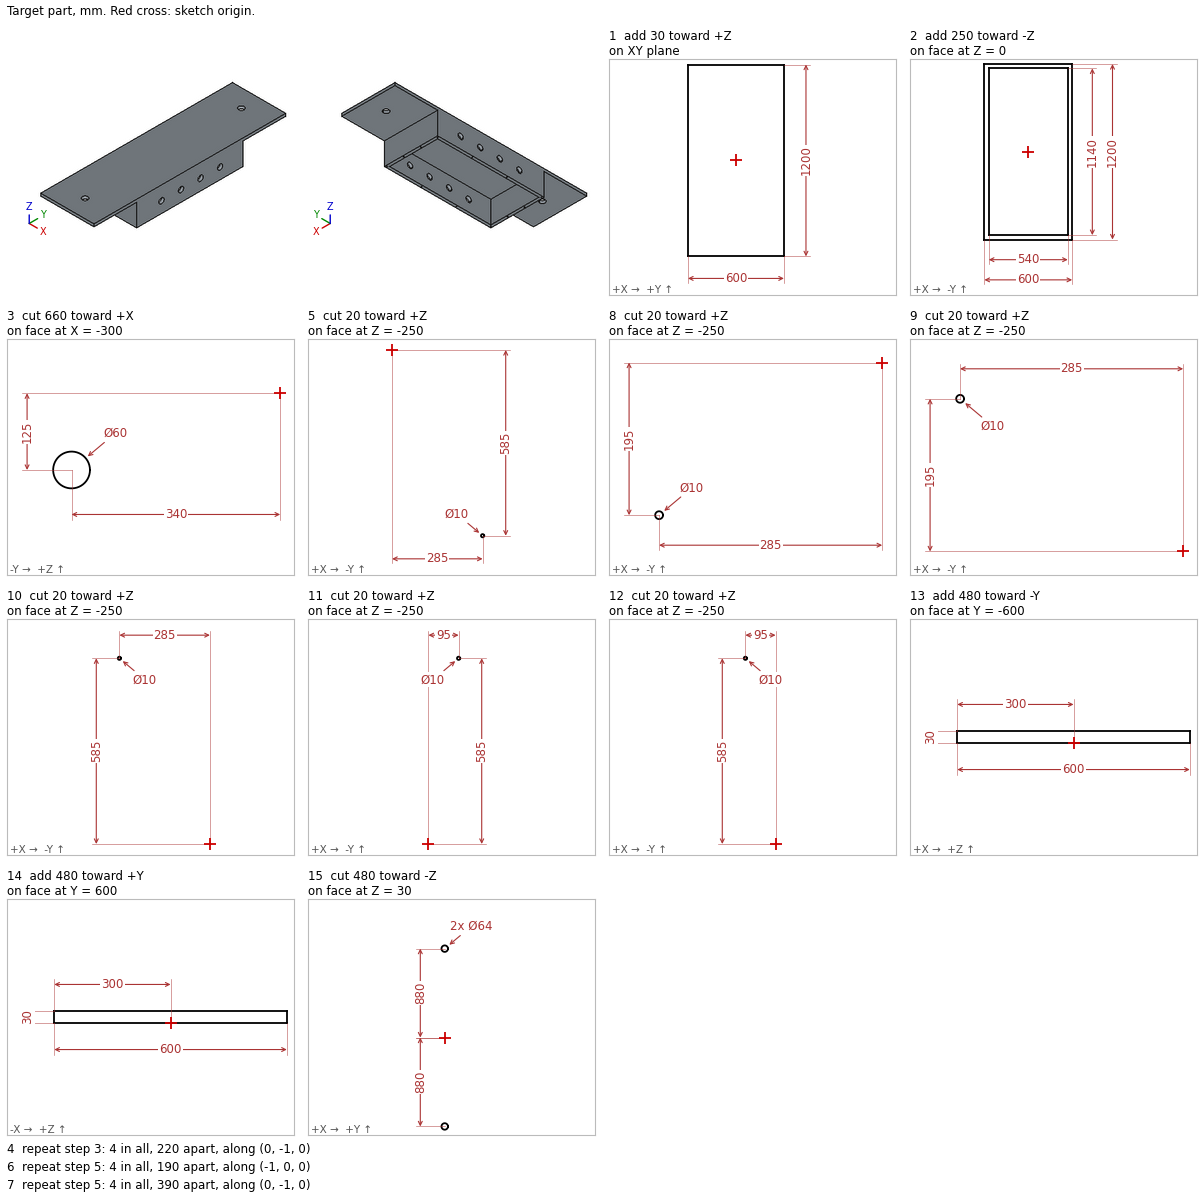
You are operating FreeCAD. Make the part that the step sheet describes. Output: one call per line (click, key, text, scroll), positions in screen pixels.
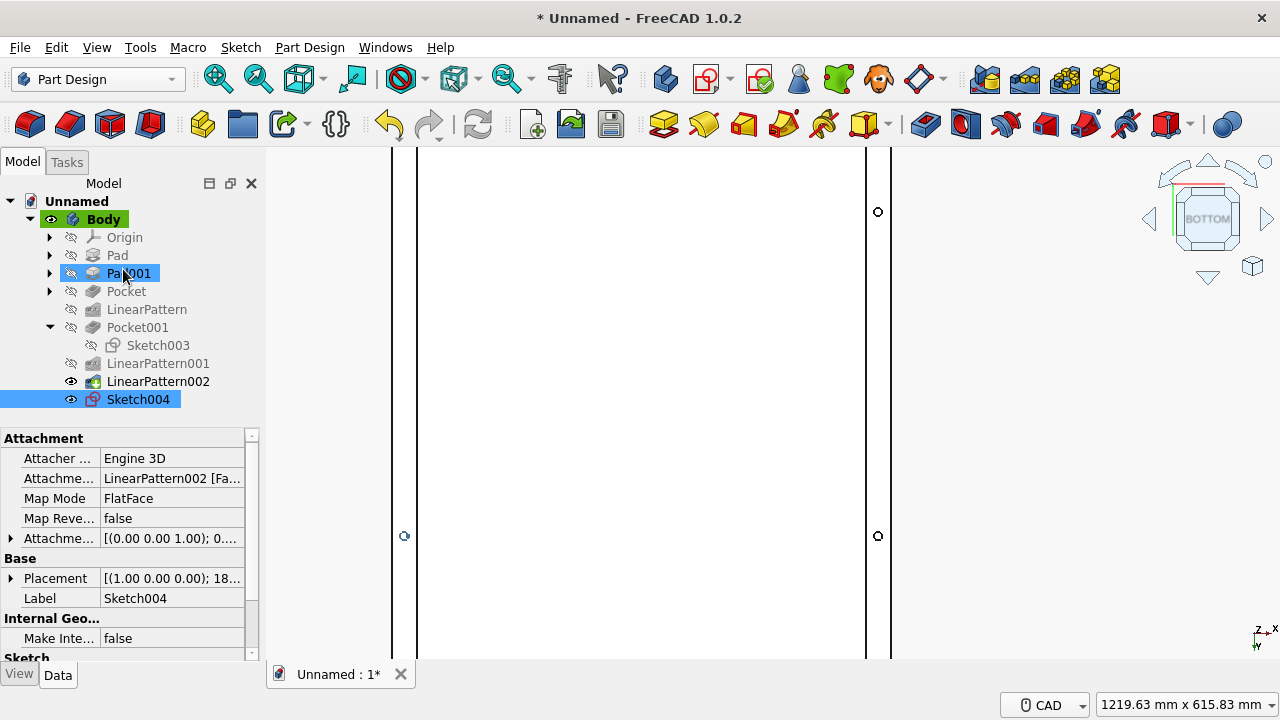
click(926, 124)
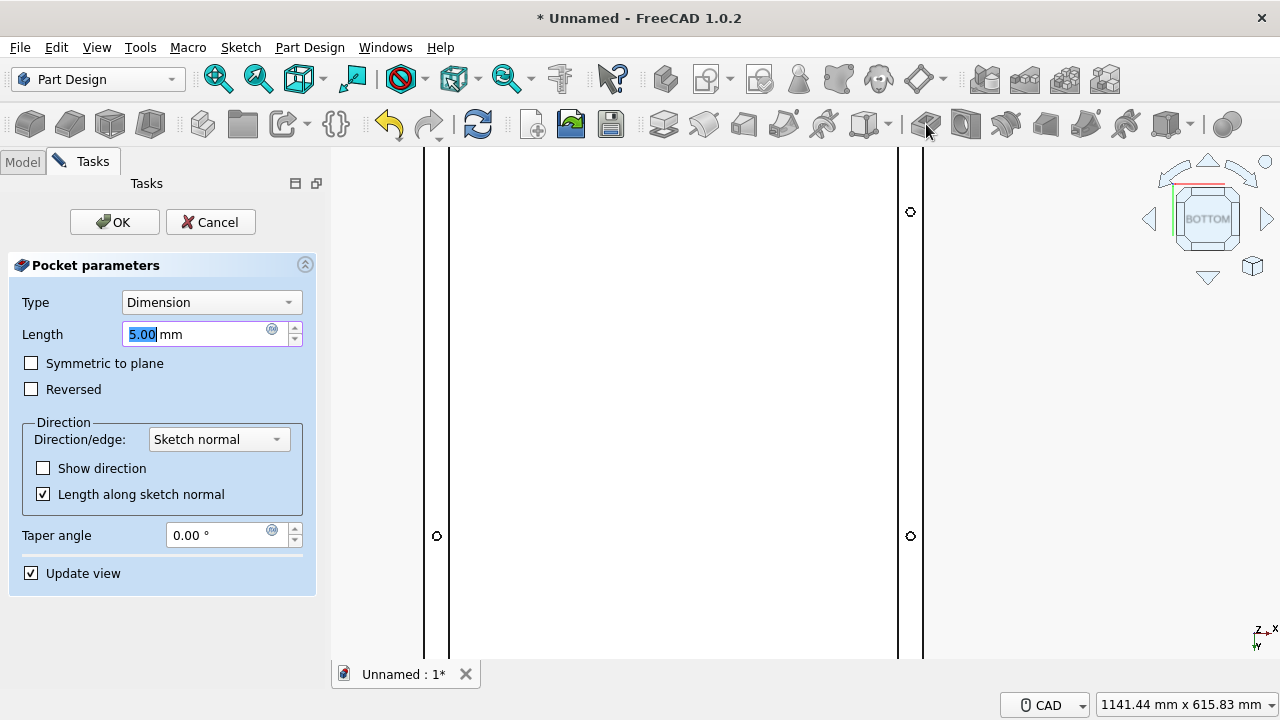
text(20)
key(Tab)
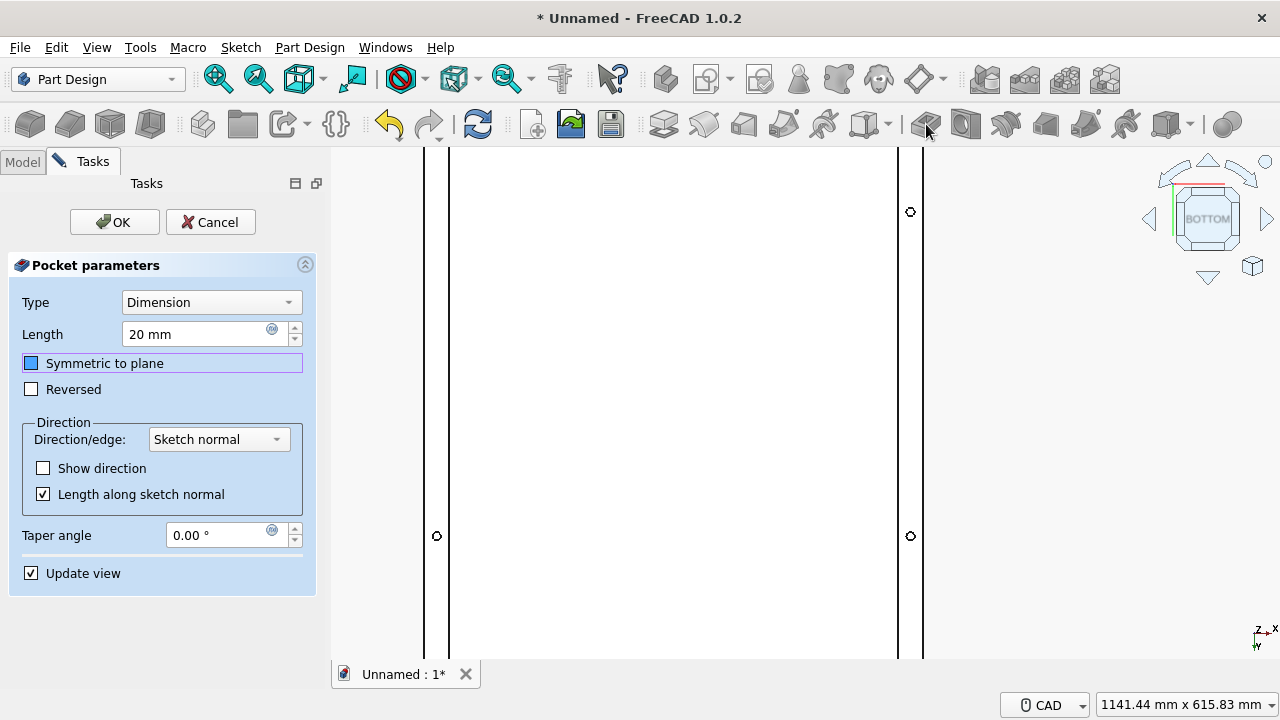
click(115, 222)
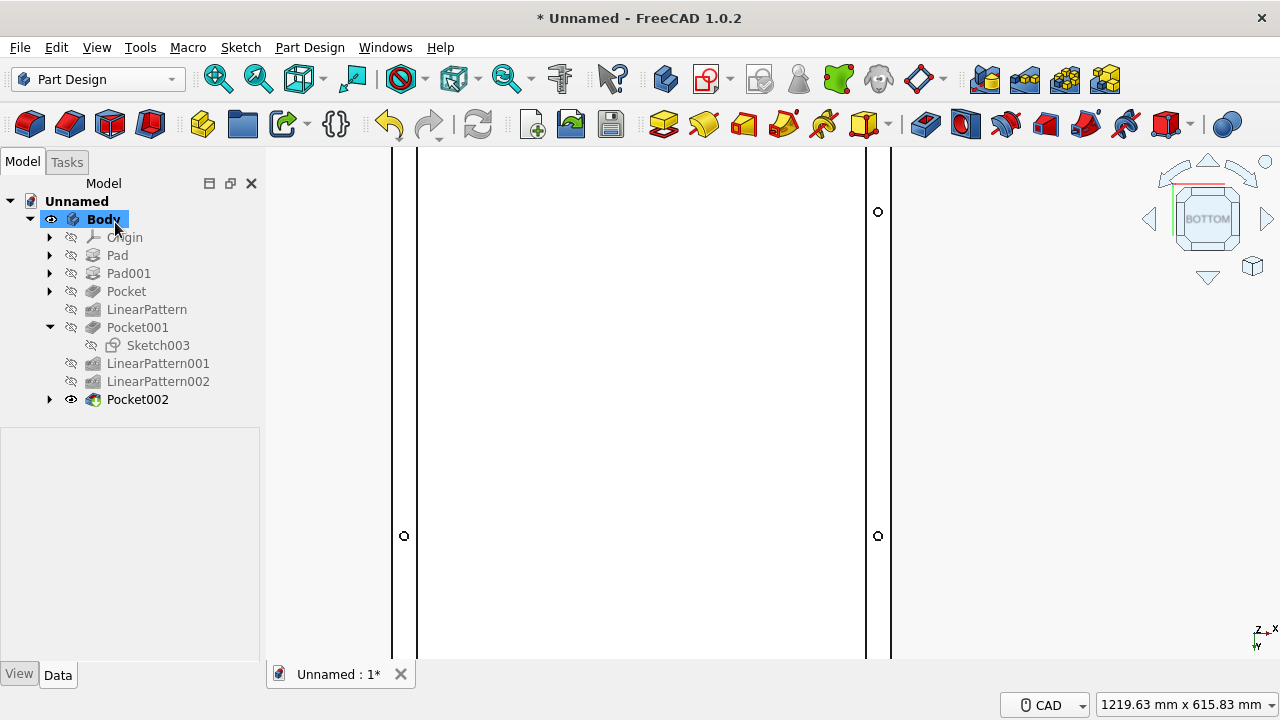
click(220, 80)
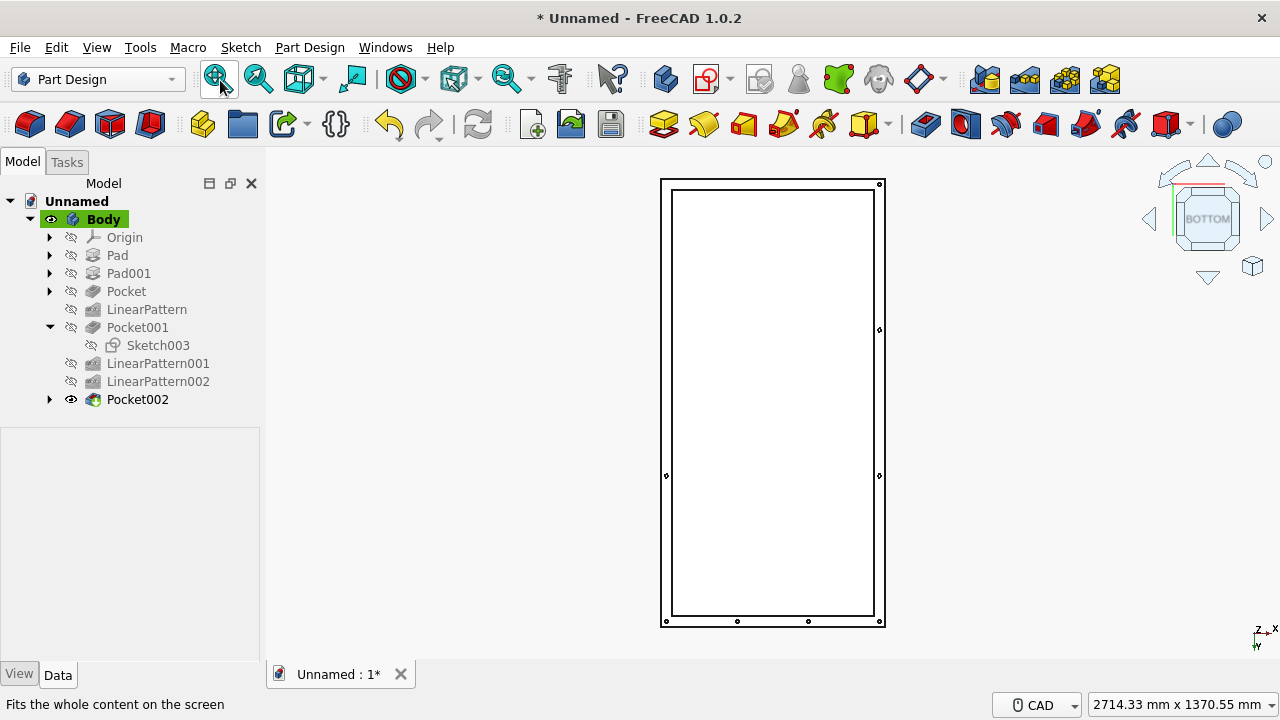
scroll(880, 426, up, 4)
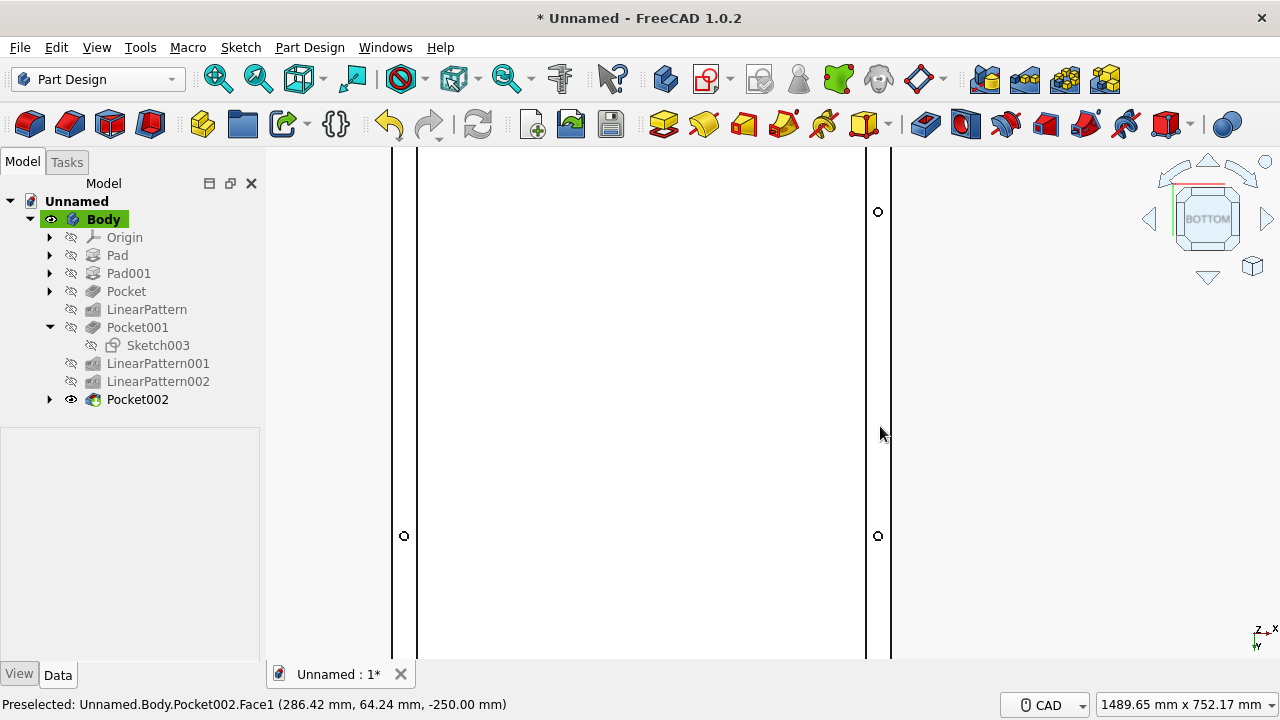
click(878, 426)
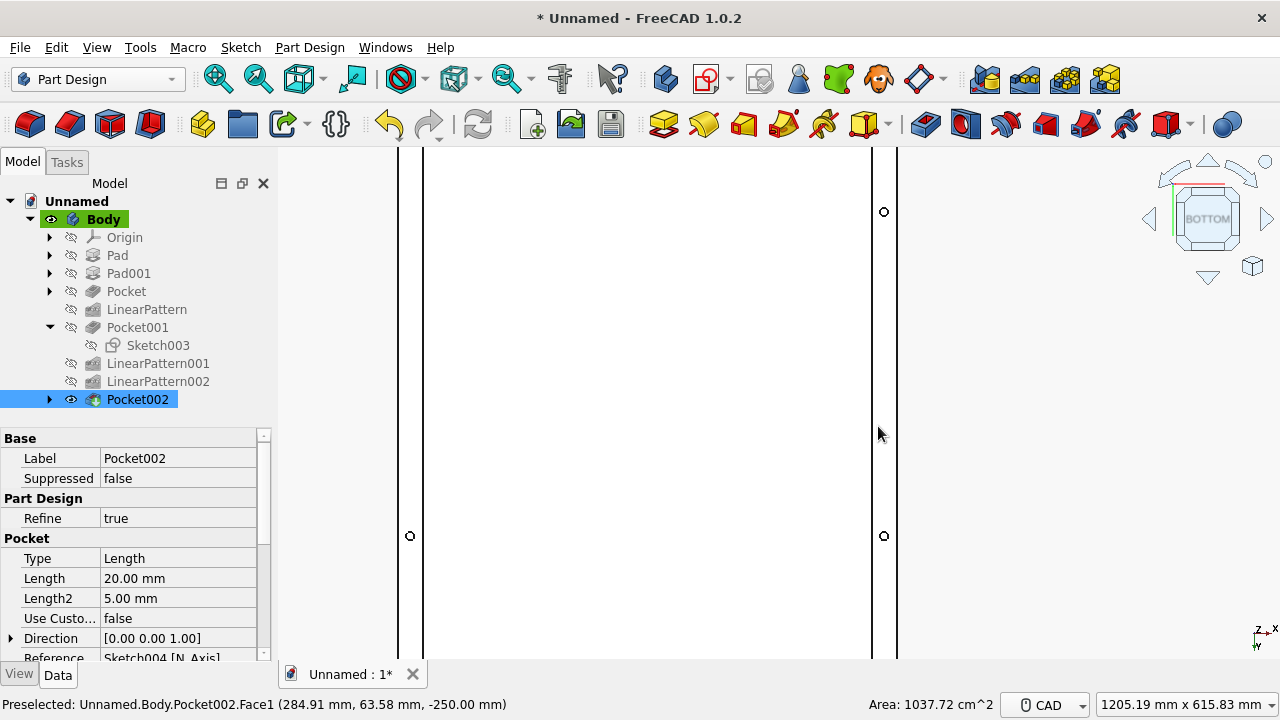
click(706, 80)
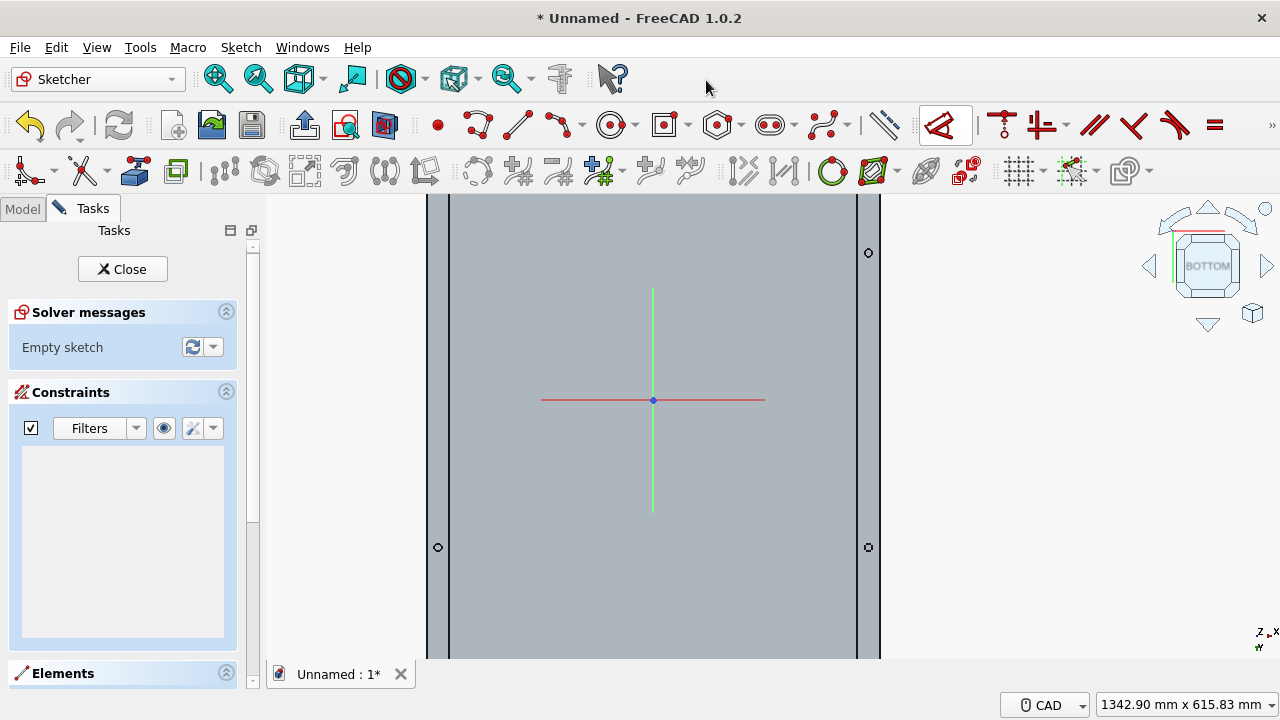
scroll(424, 244, up, 15)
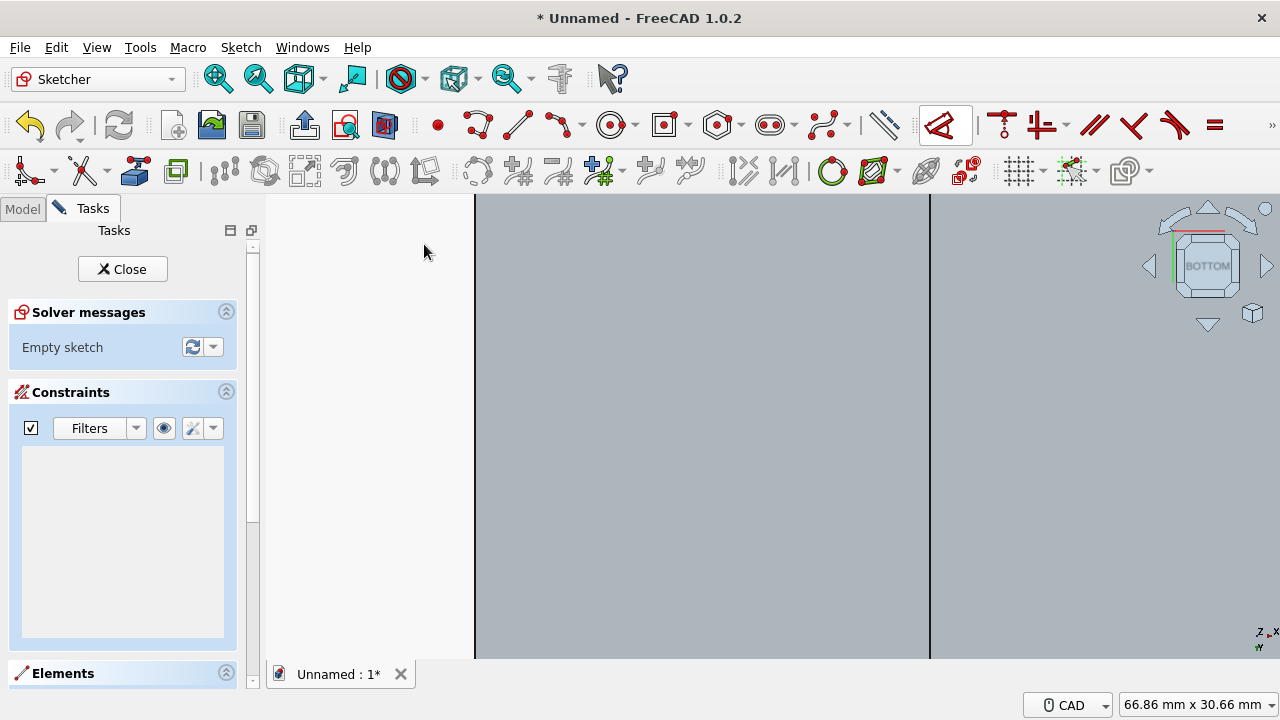
scroll(701, 420, up, 3)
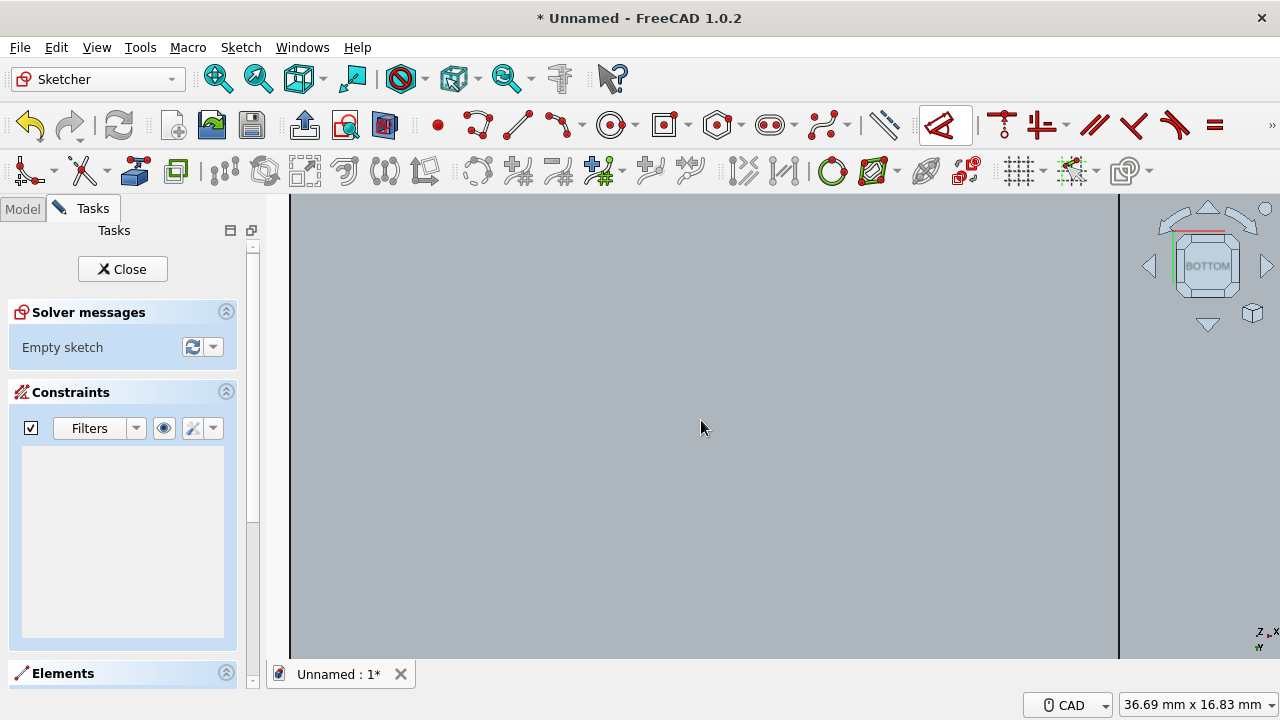
click(612, 126)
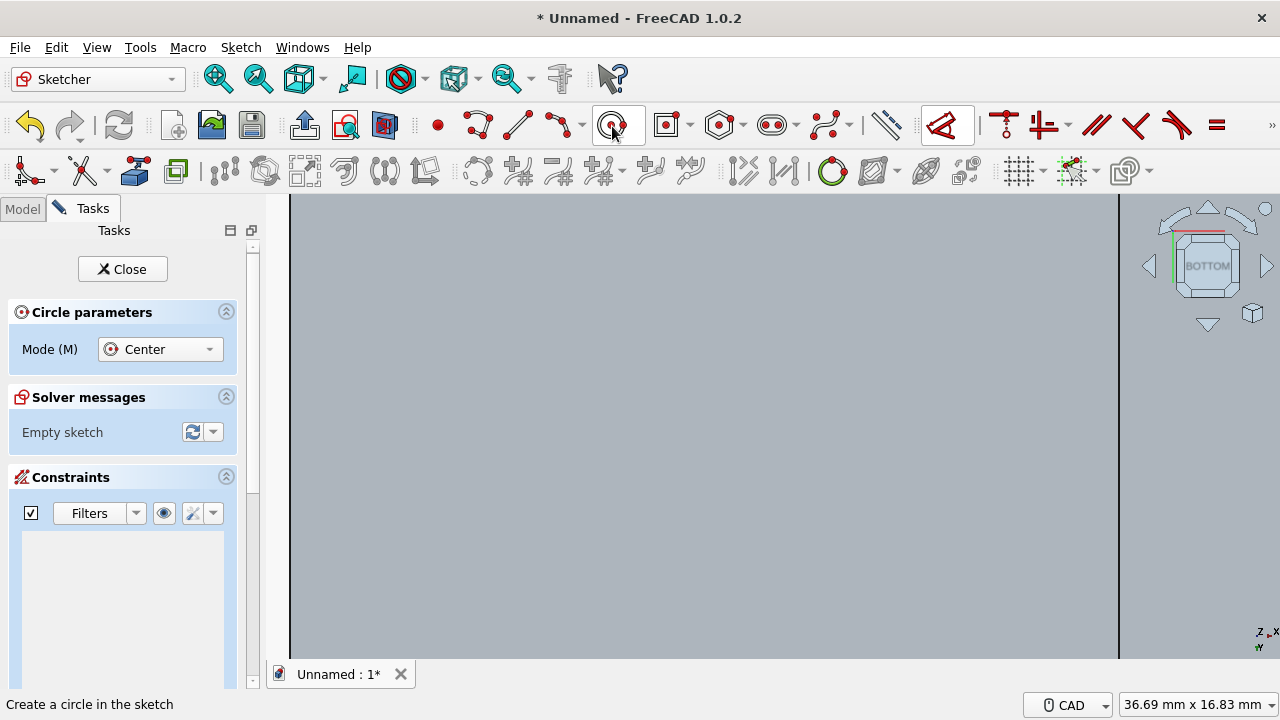
click(704, 426)
move(802, 329)